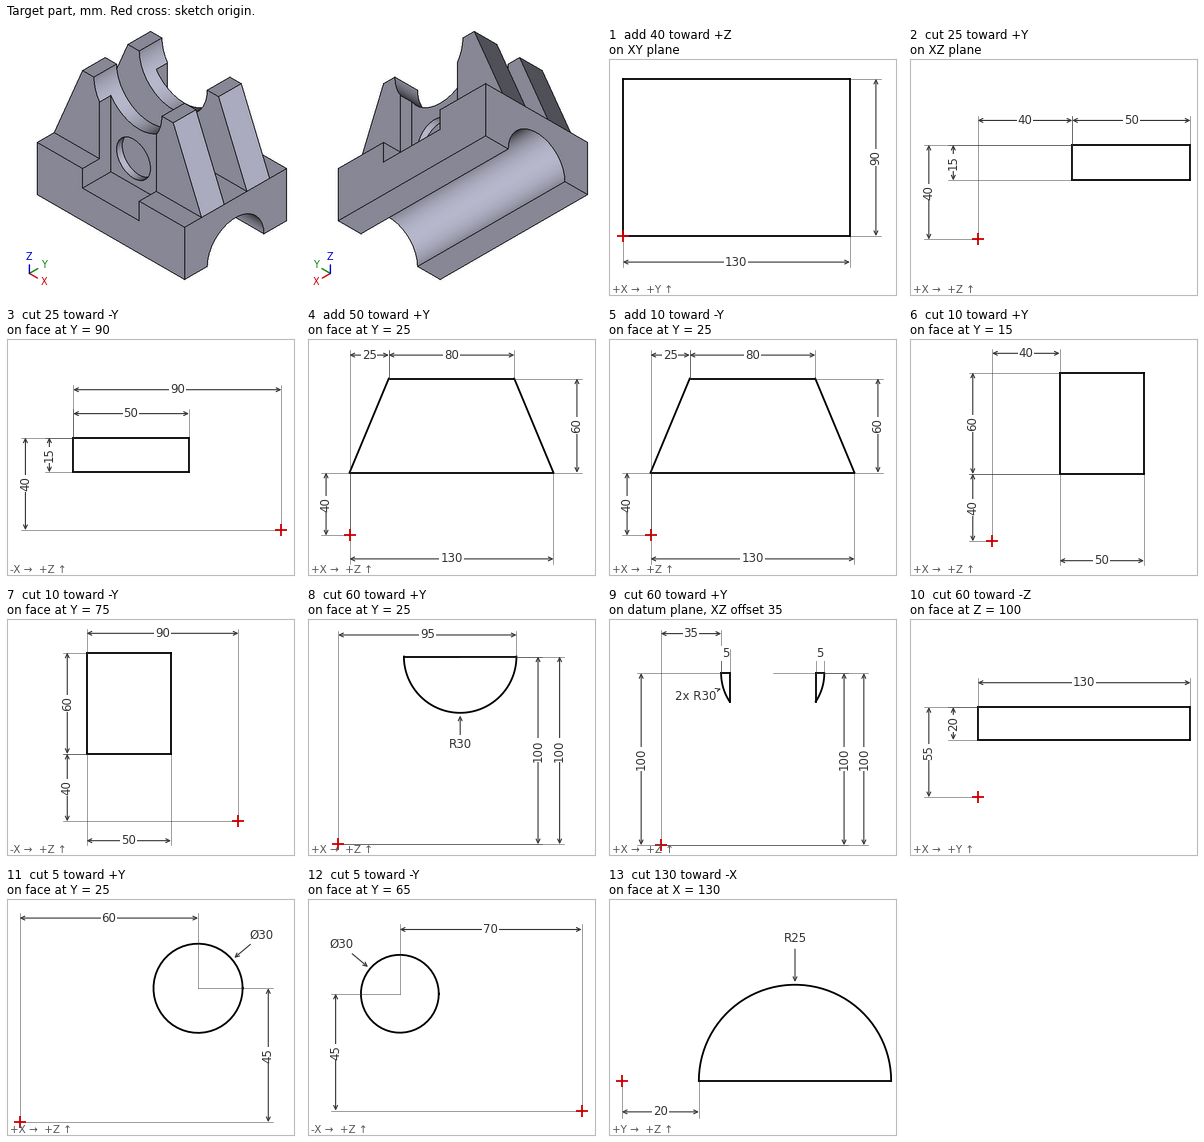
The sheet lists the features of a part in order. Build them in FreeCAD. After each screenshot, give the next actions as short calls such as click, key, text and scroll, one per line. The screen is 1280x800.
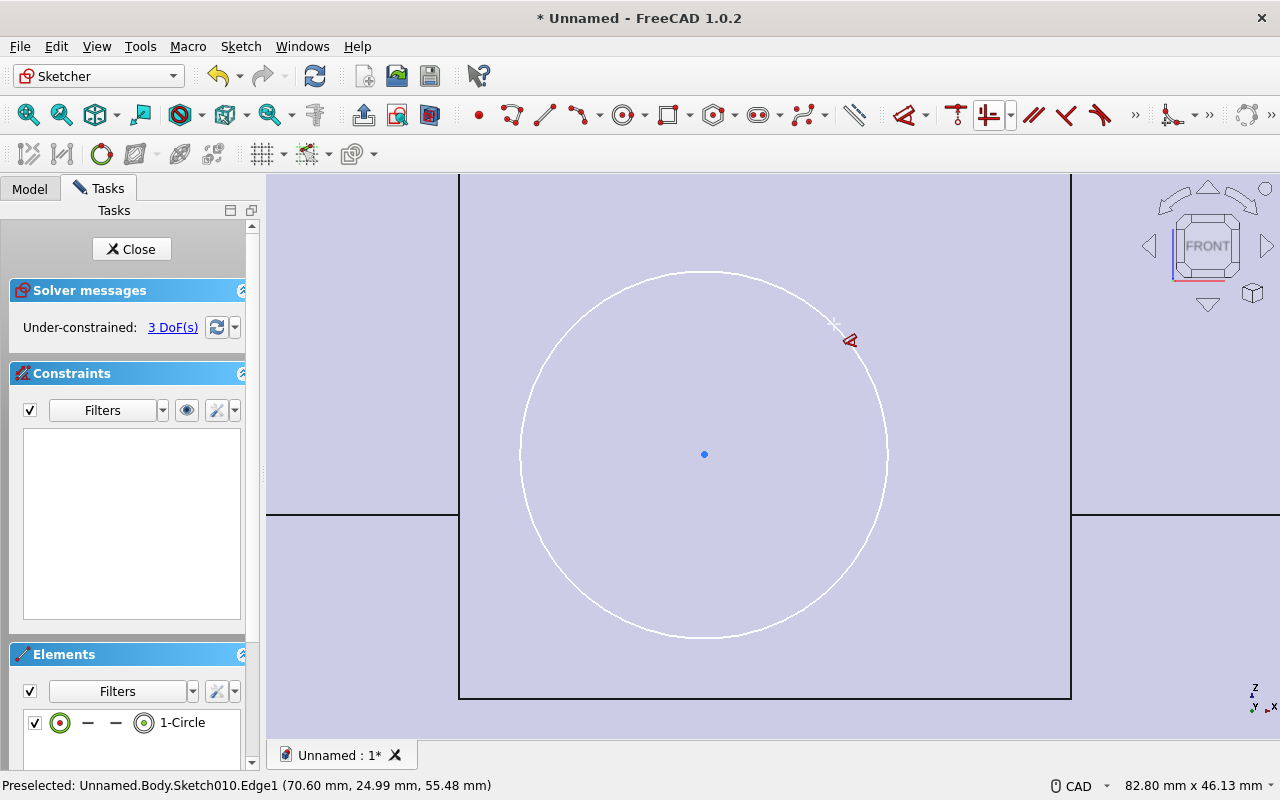
click(834, 325)
click(857, 302)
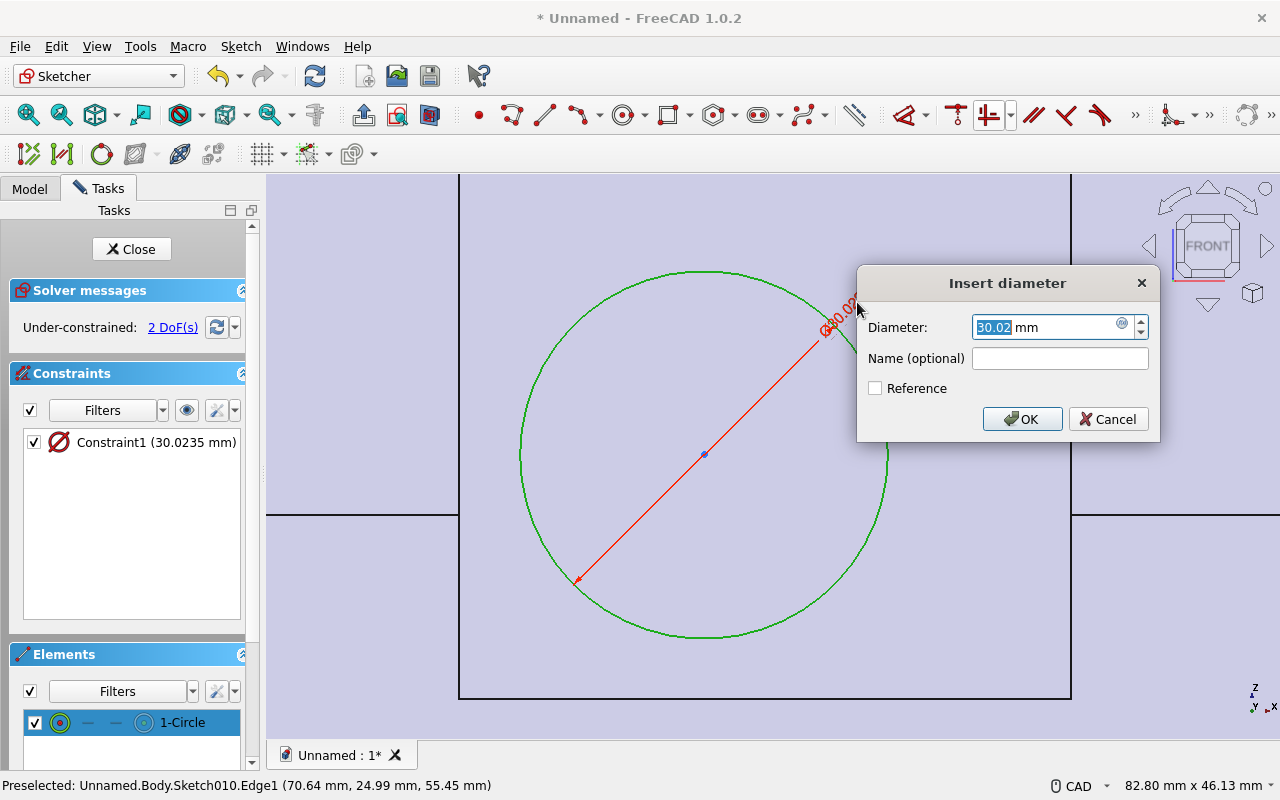
text(30)
key(Return)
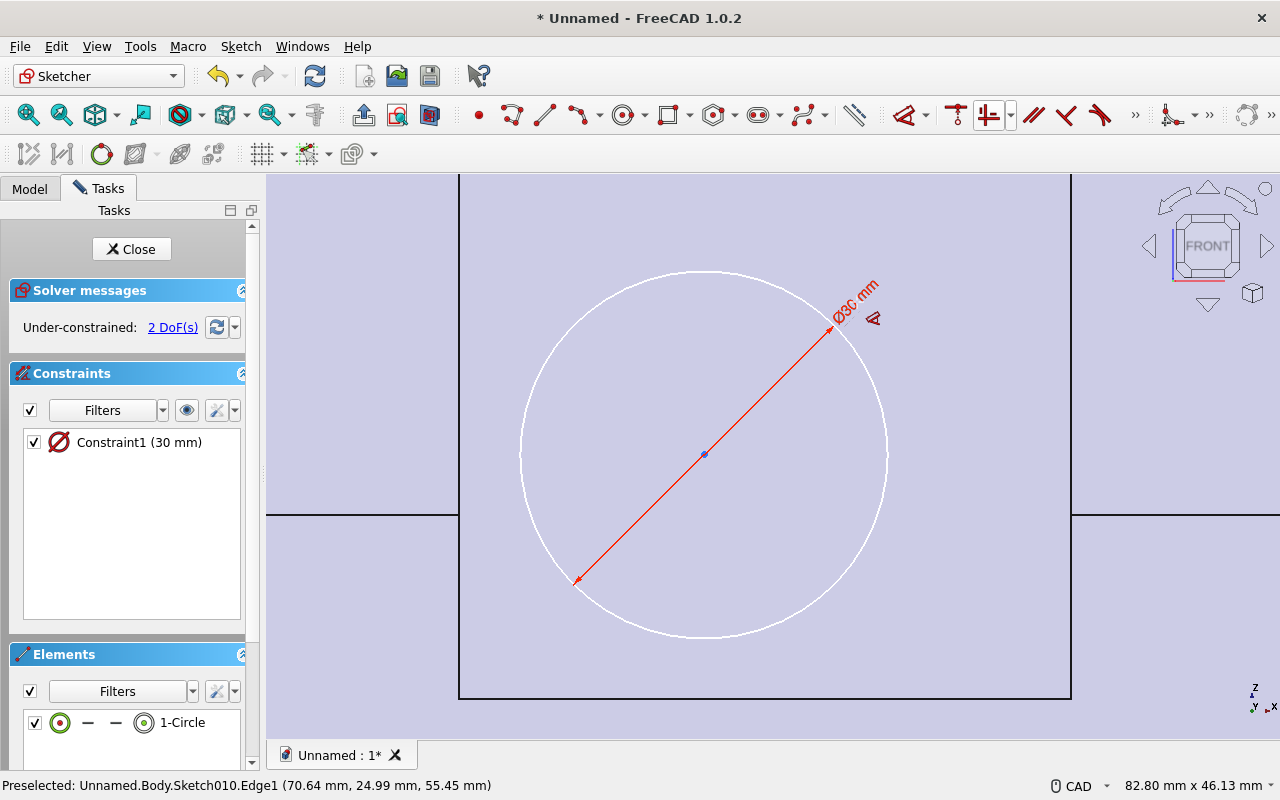
click(704, 455)
click(499, 421)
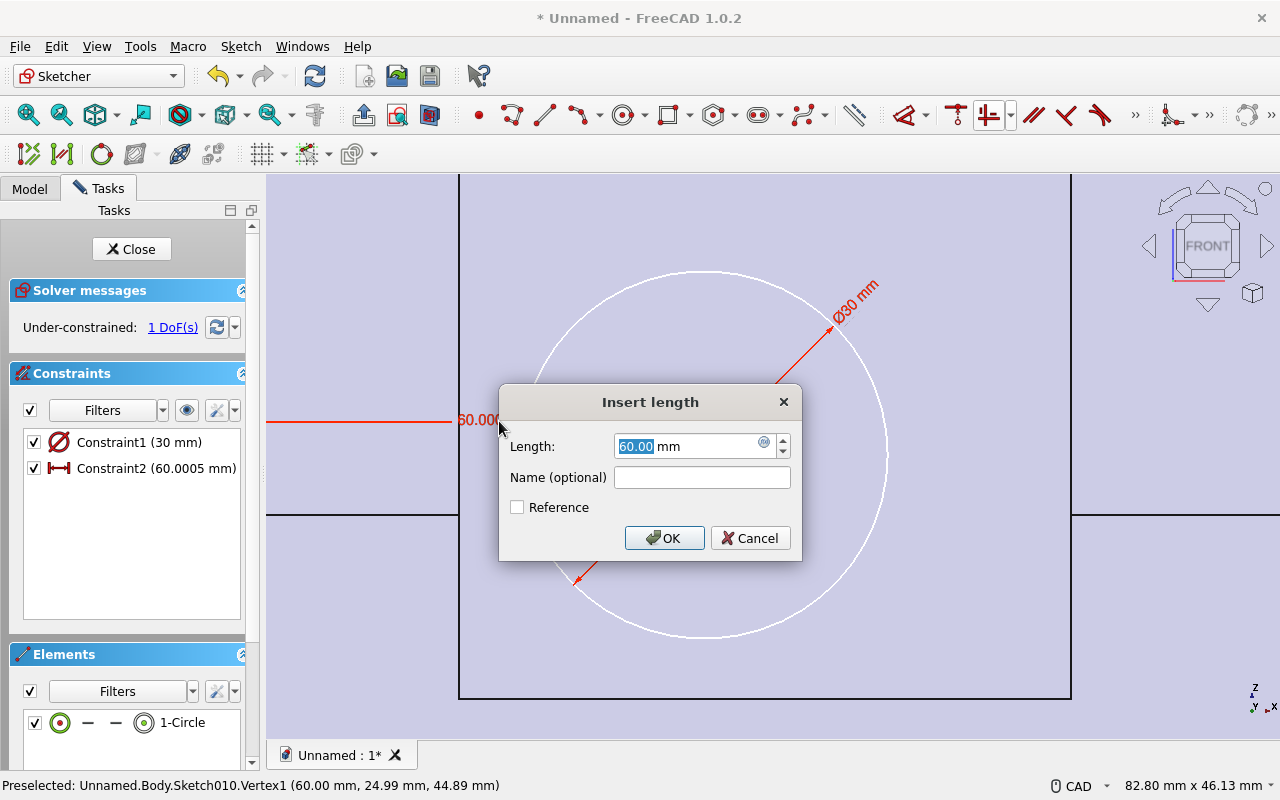
text(60)
key(Return)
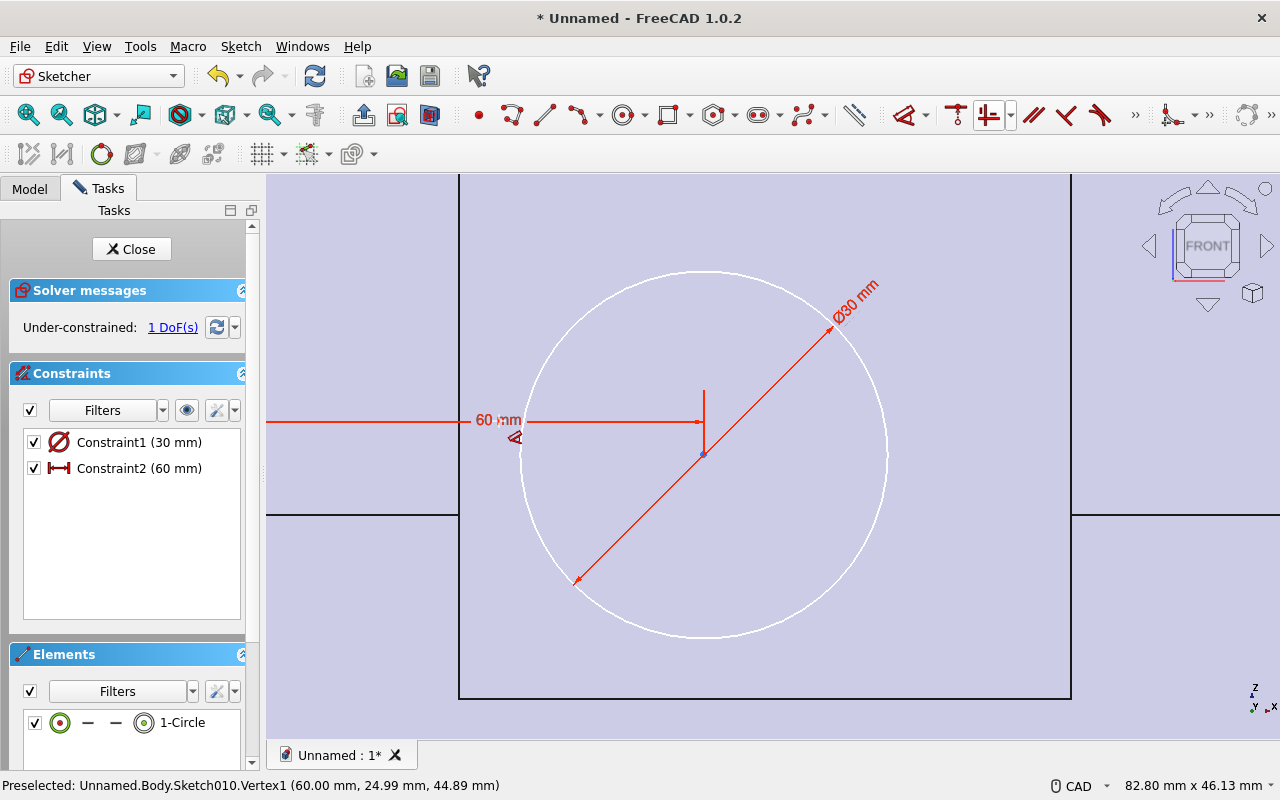
click(704, 455)
click(738, 583)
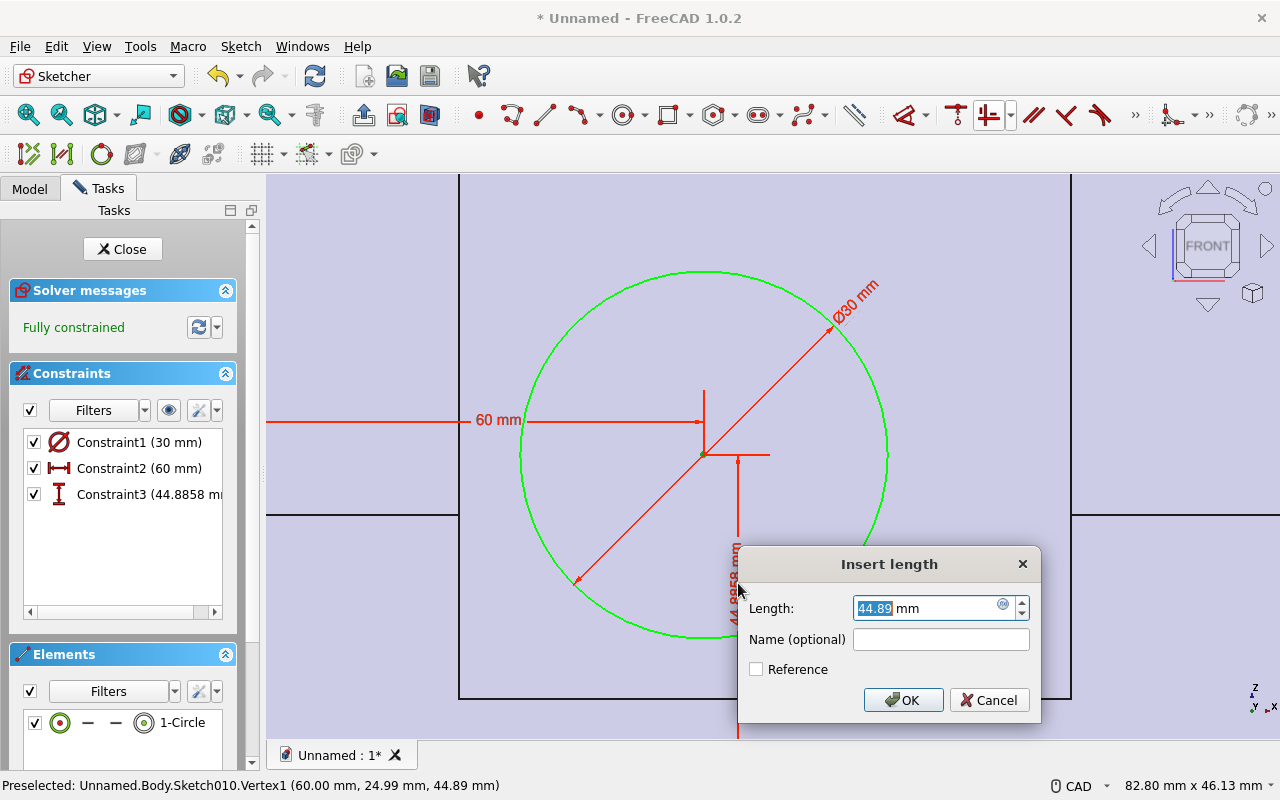
text(45)
key(Return)
key(Escape)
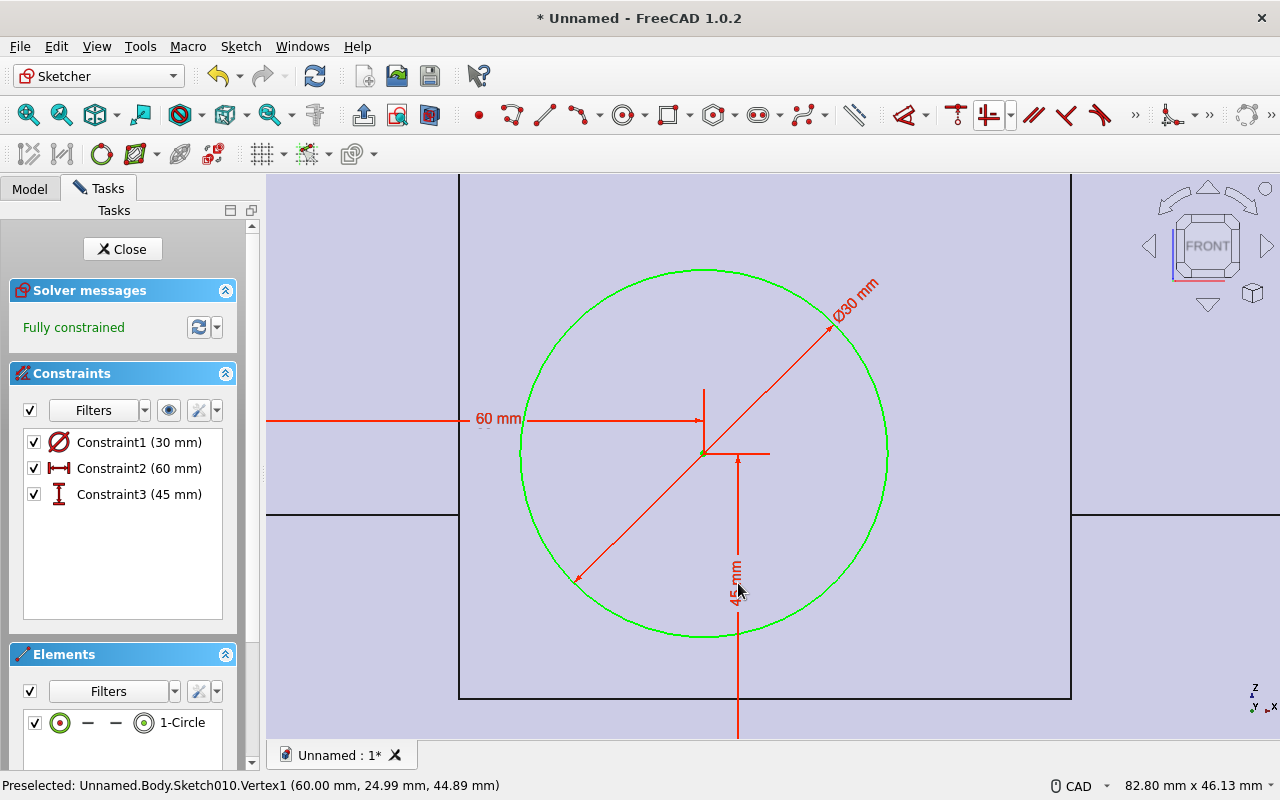
click(123, 249)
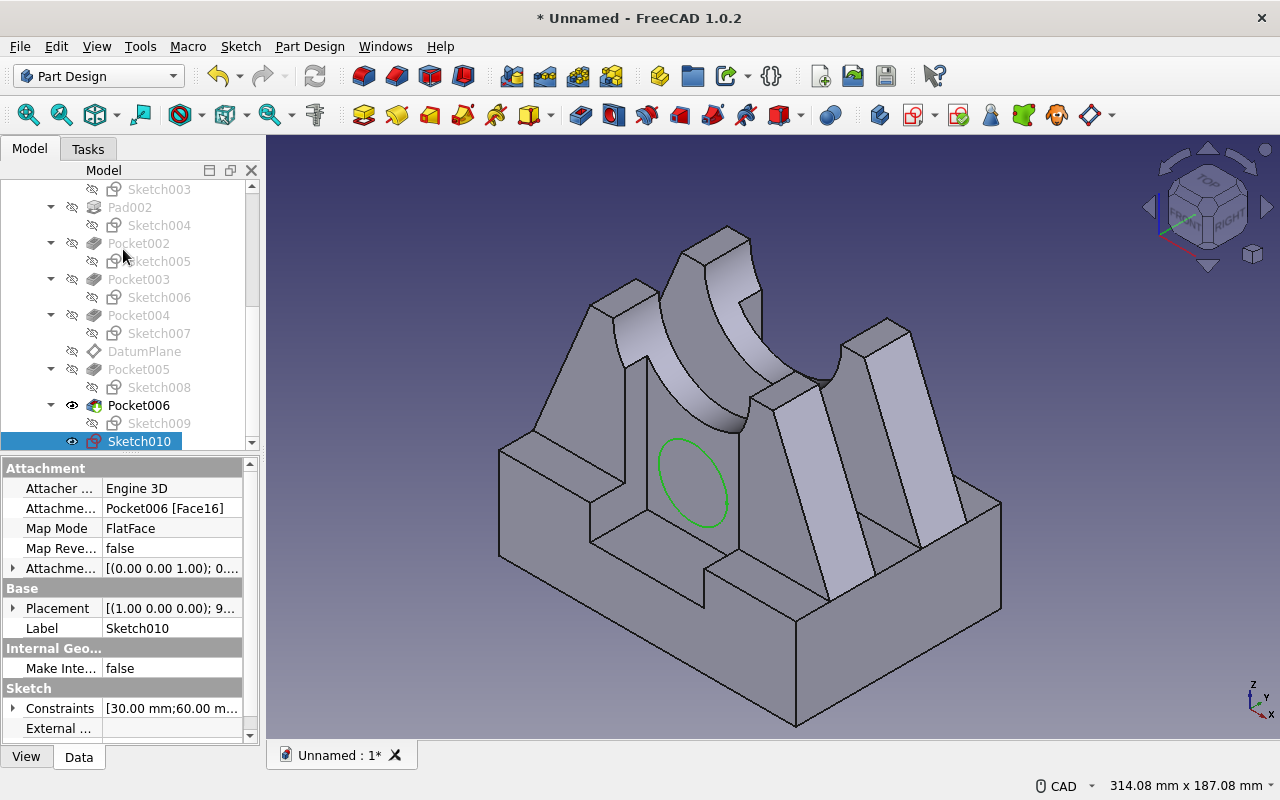
click(581, 116)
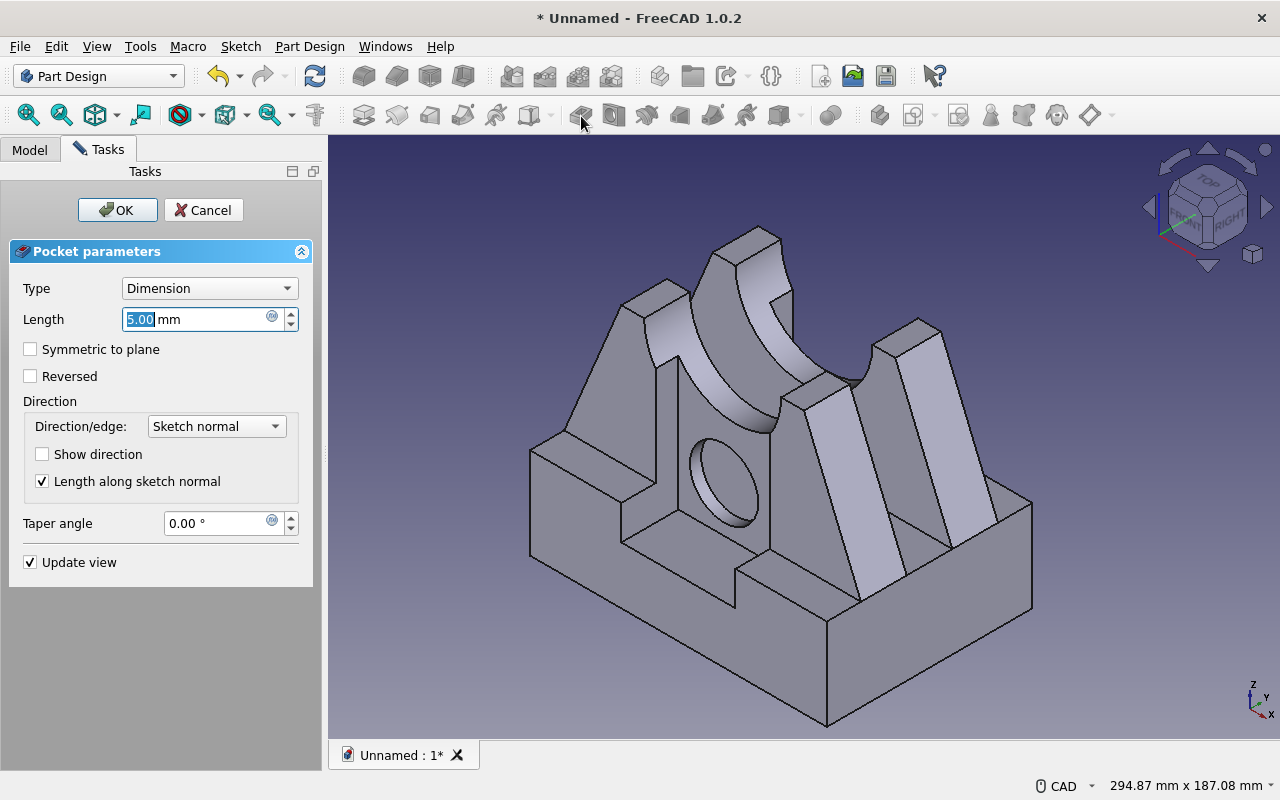
text(5)
key(Tab)